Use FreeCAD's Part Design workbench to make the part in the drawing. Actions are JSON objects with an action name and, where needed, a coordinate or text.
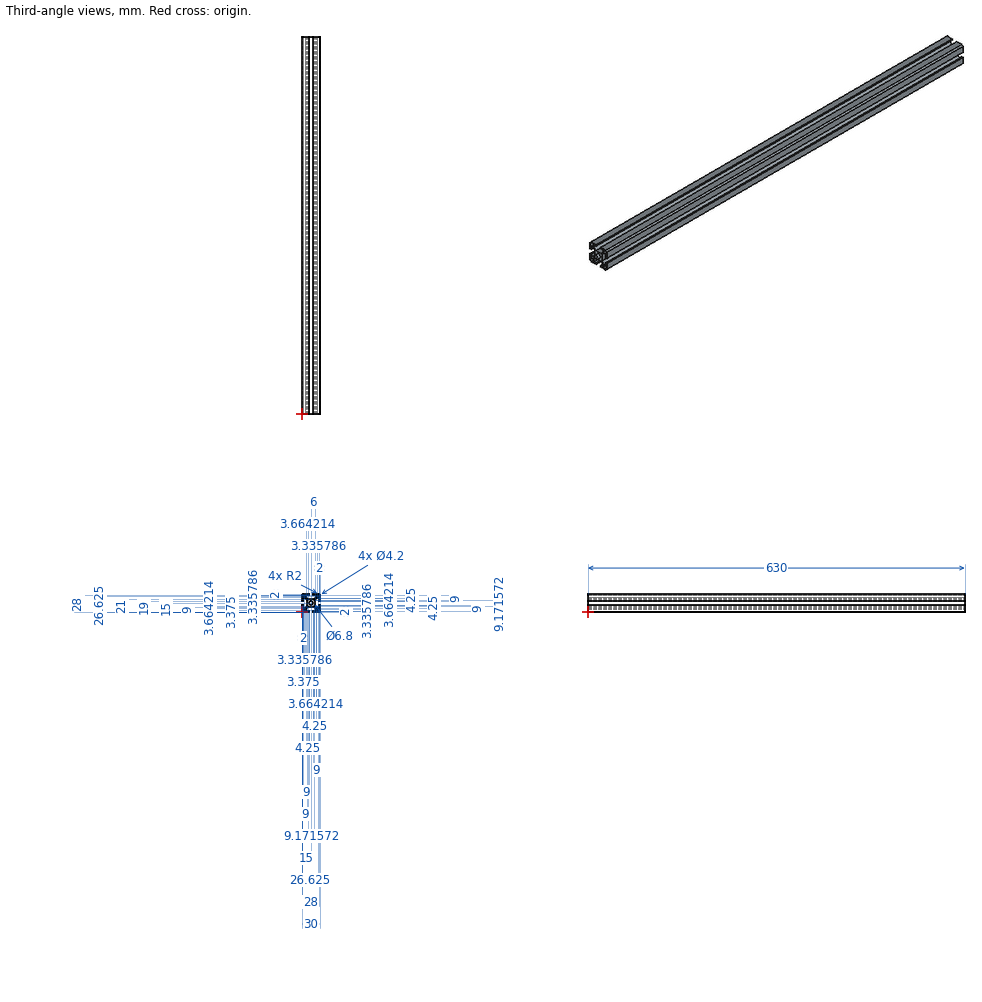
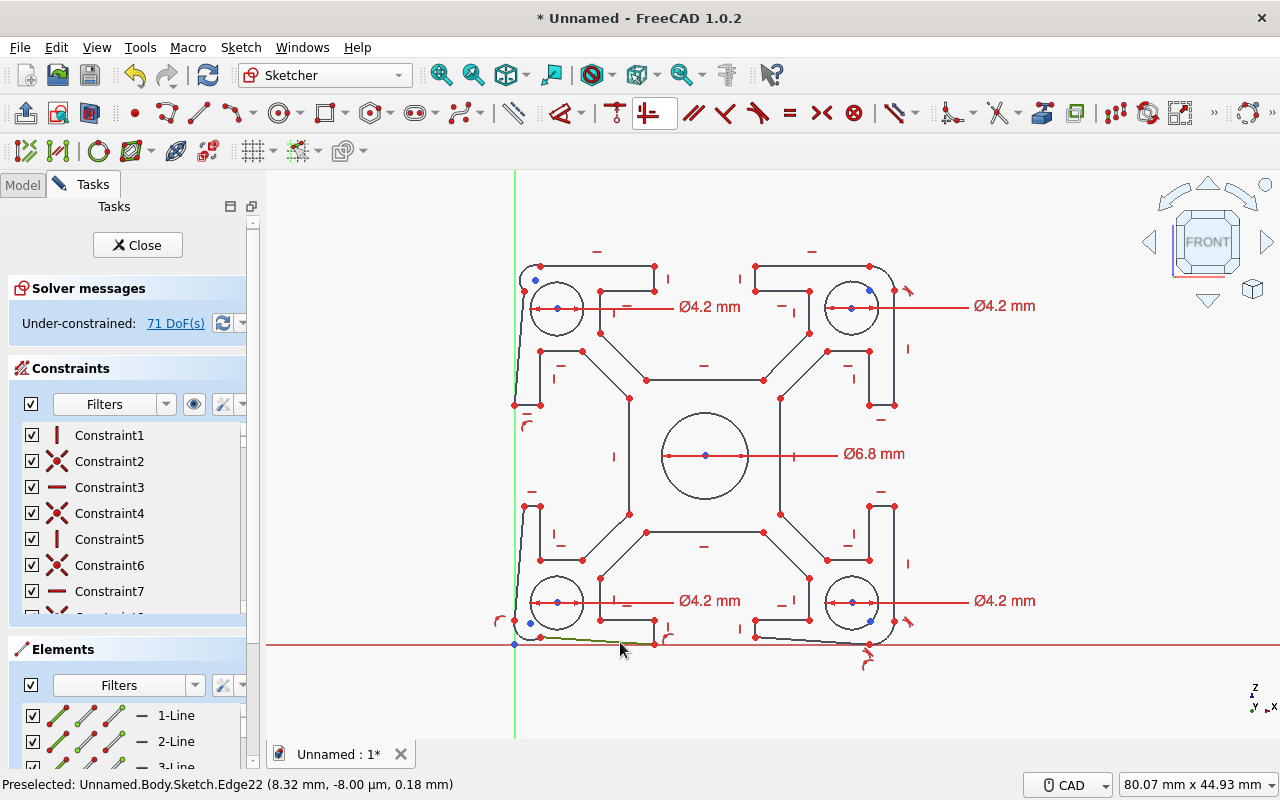
{"action": "left_click", "coordinate": [516, 632]}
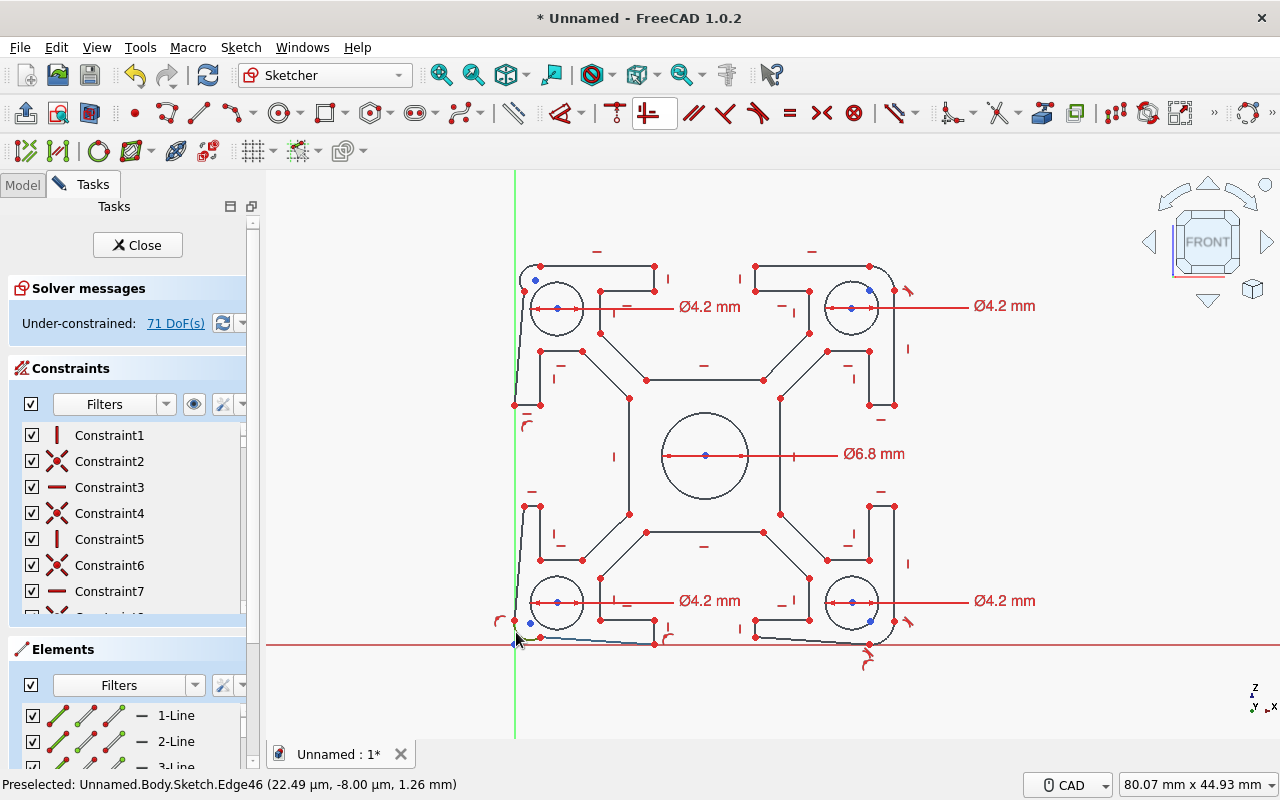
{"action": "left_click", "coordinate": [758, 114]}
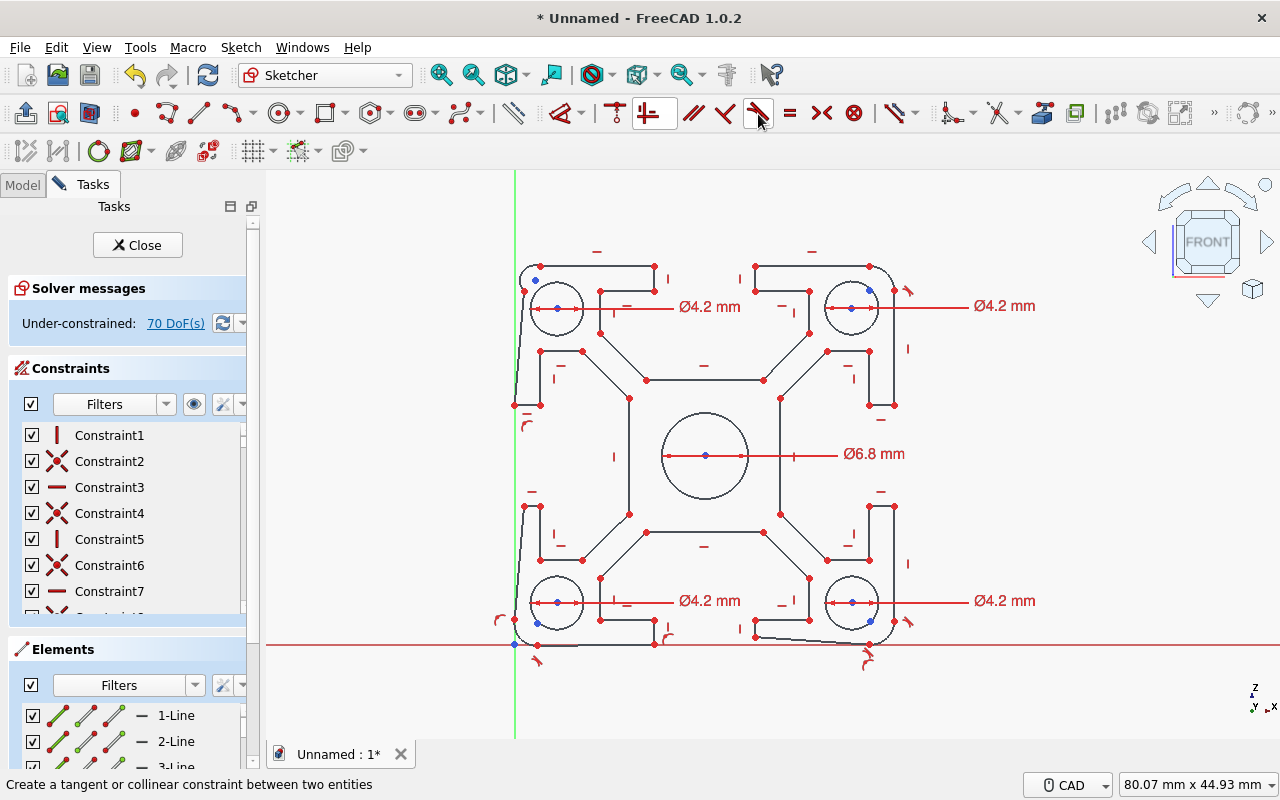
{"action": "left_click", "coordinate": [517, 586]}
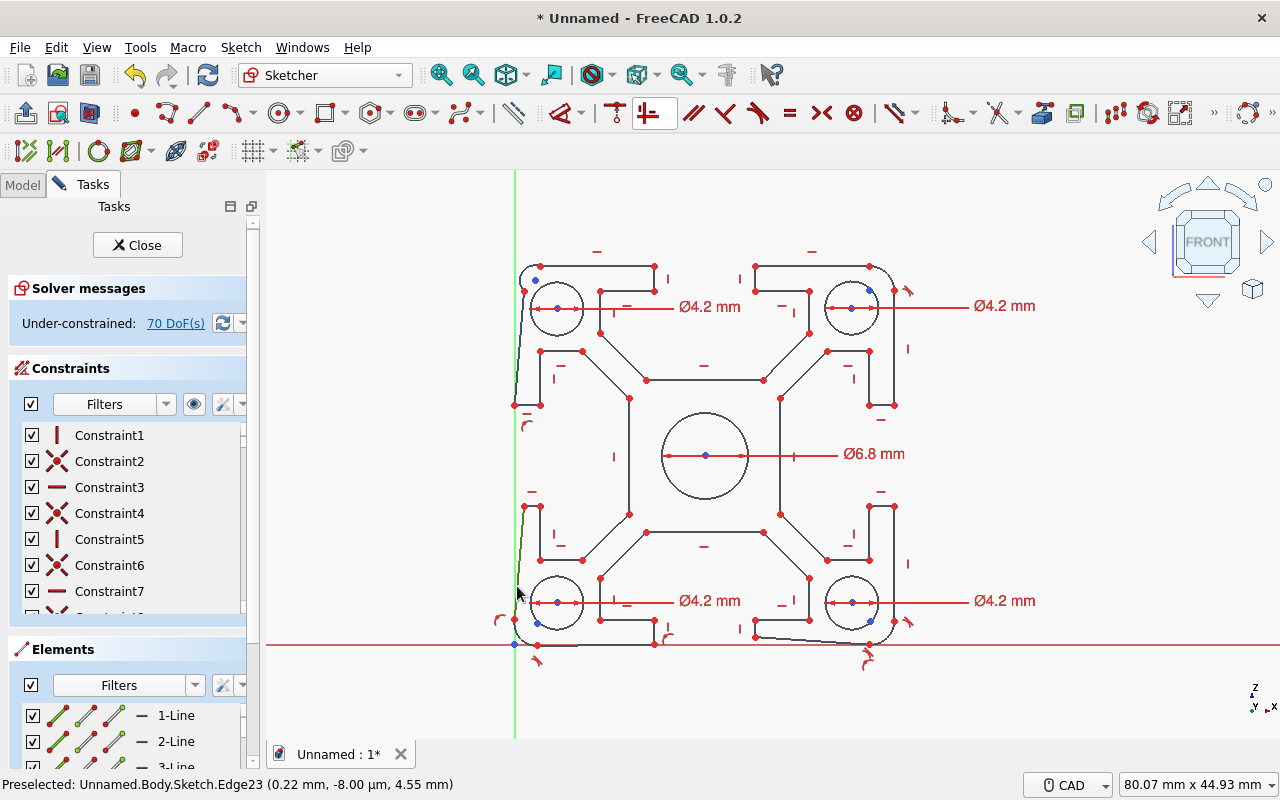
{"action": "left_click", "coordinate": [516, 631]}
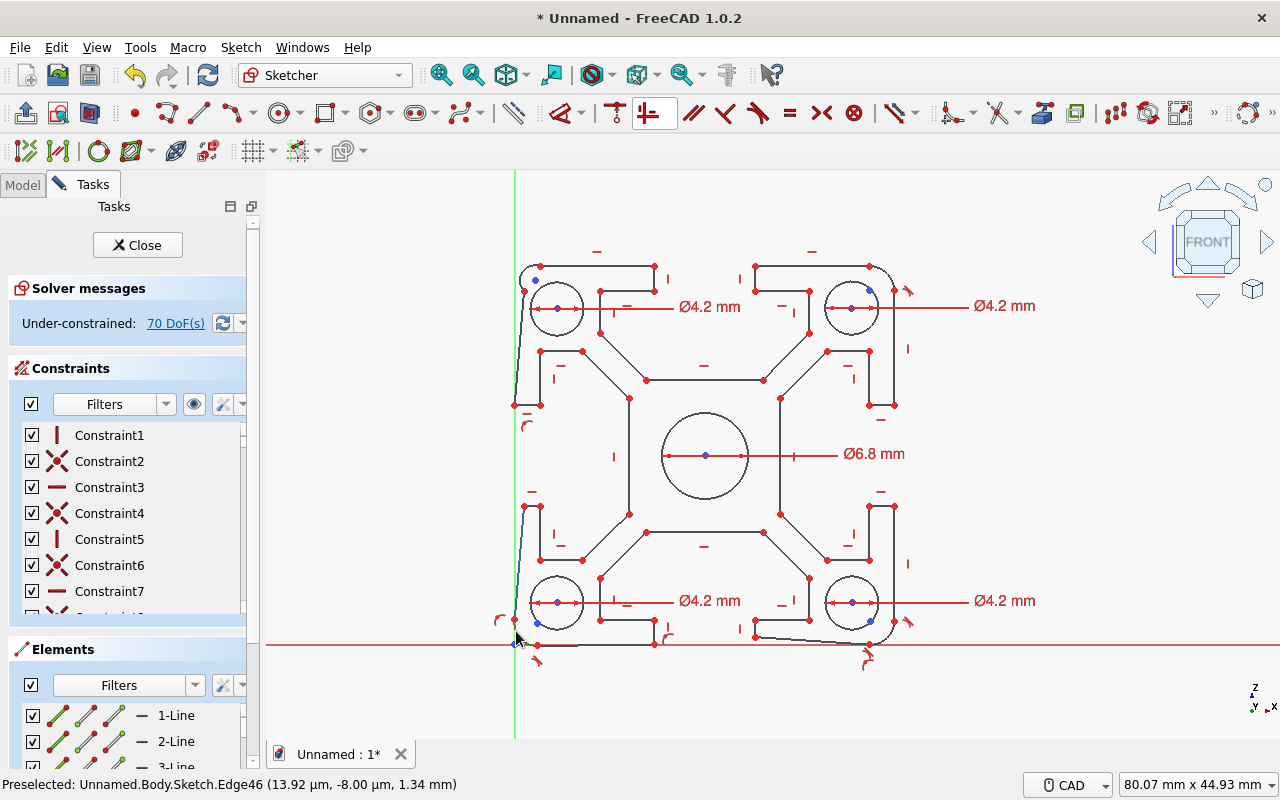
{"action": "key", "text": "t"}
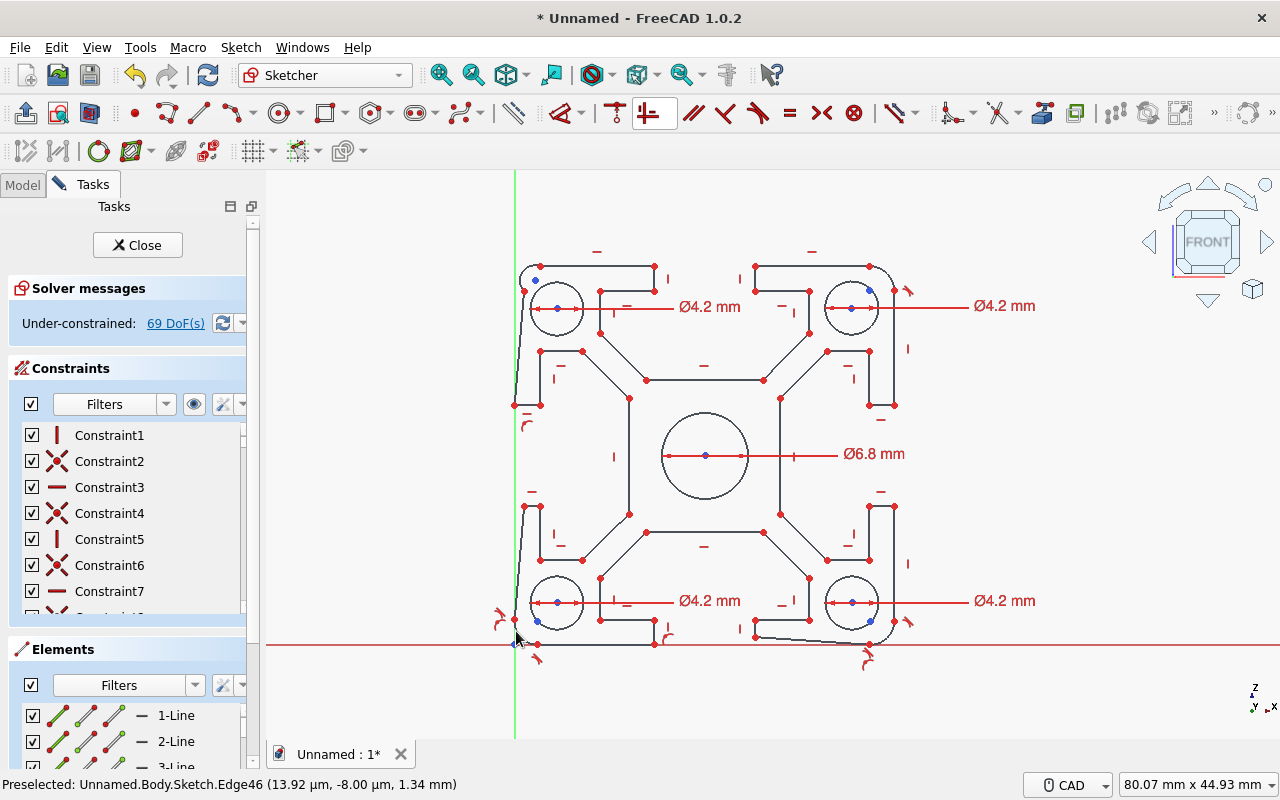
{"action": "left_click", "coordinate": [517, 371]}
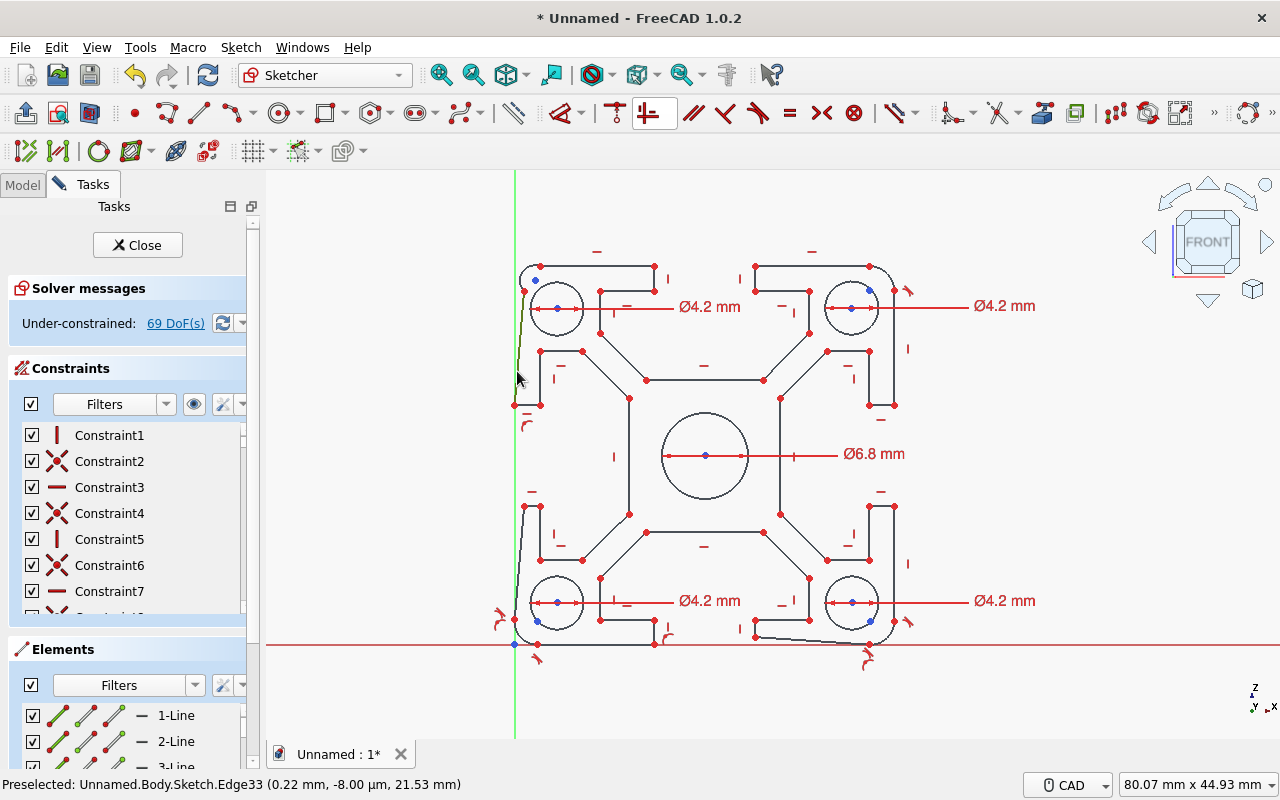
{"action": "left_click", "coordinate": [528, 267]}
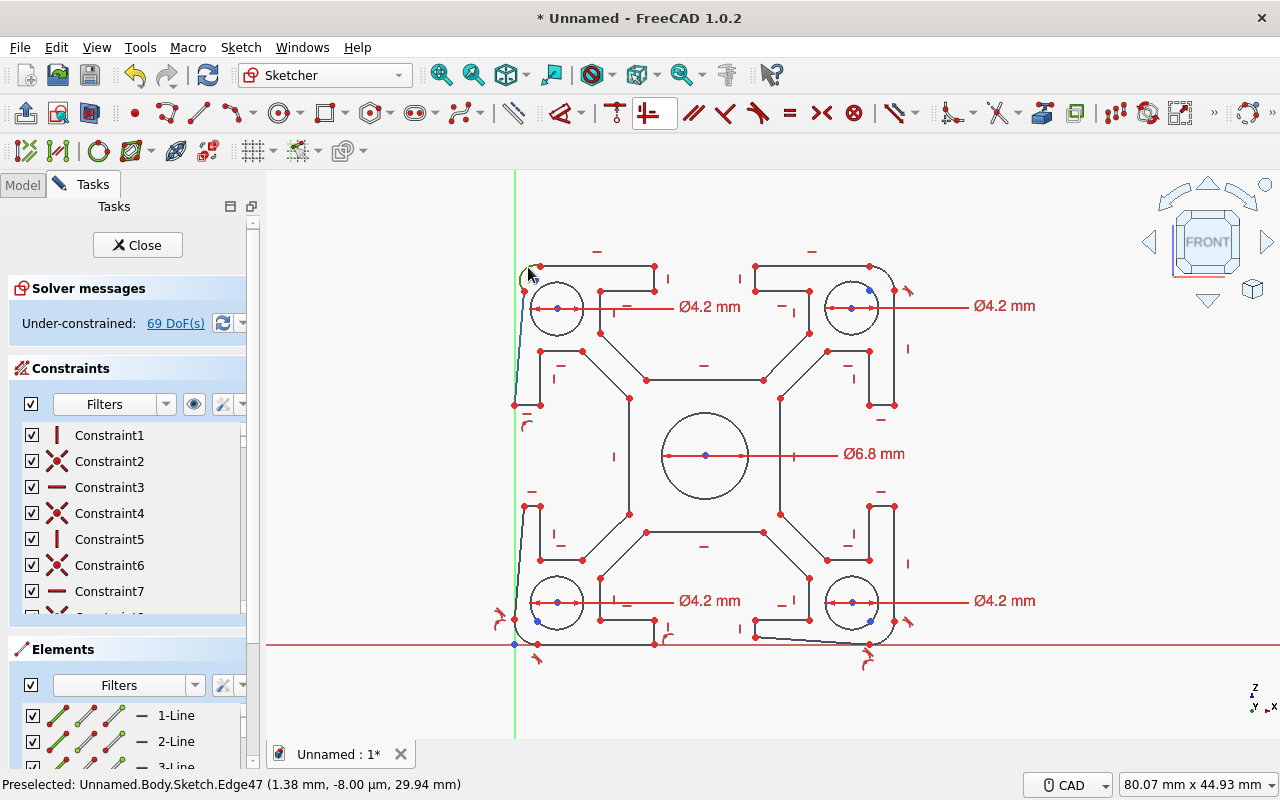
{"action": "key", "text": "t"}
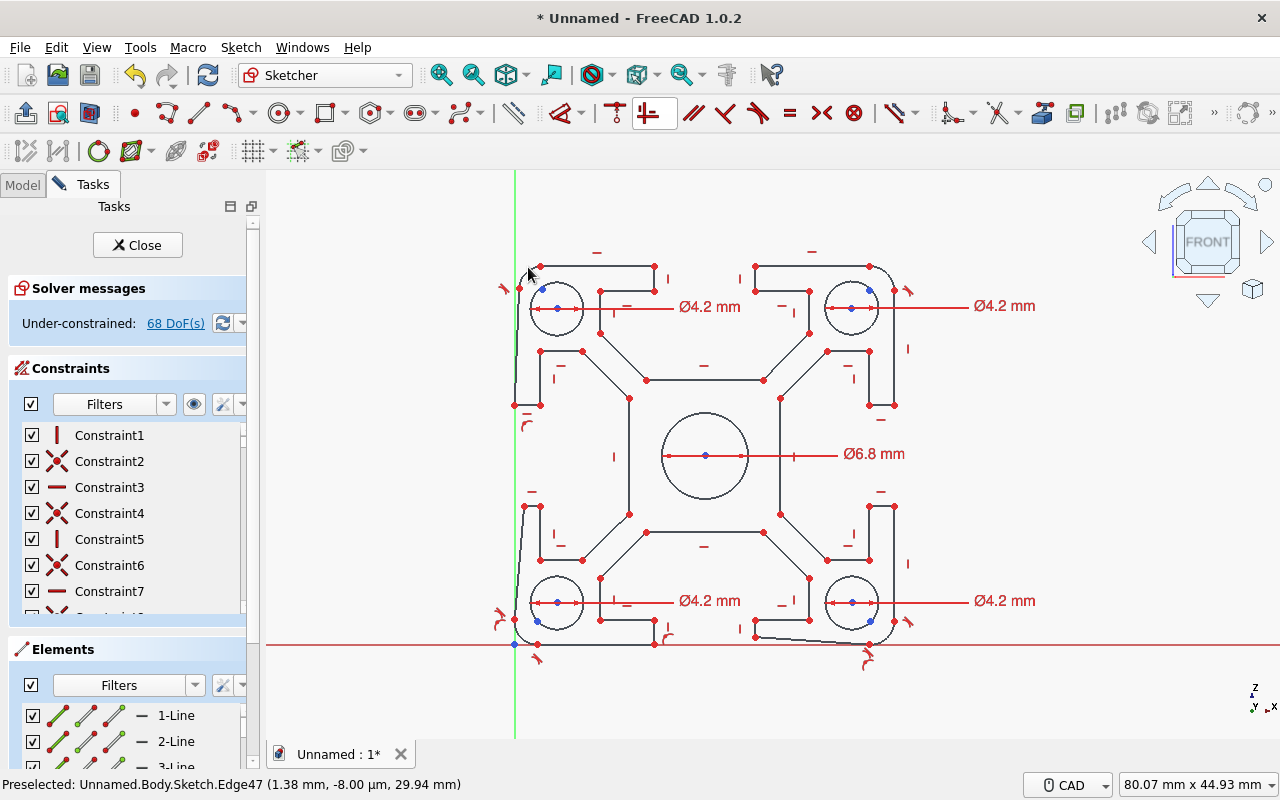
{"action": "left_click", "coordinate": [575, 266]}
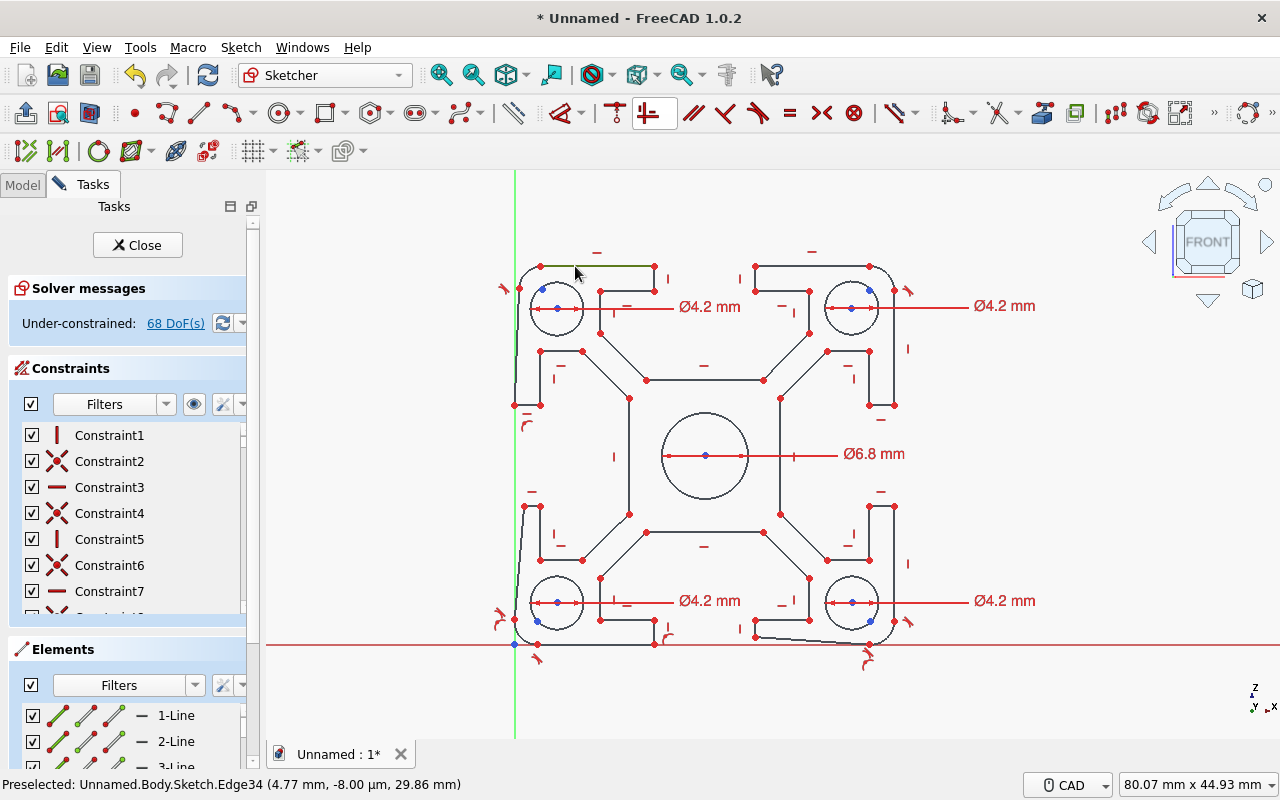
{"action": "scroll", "coordinate": [531, 269], "scroll_direction": "up", "scroll_amount": 2}